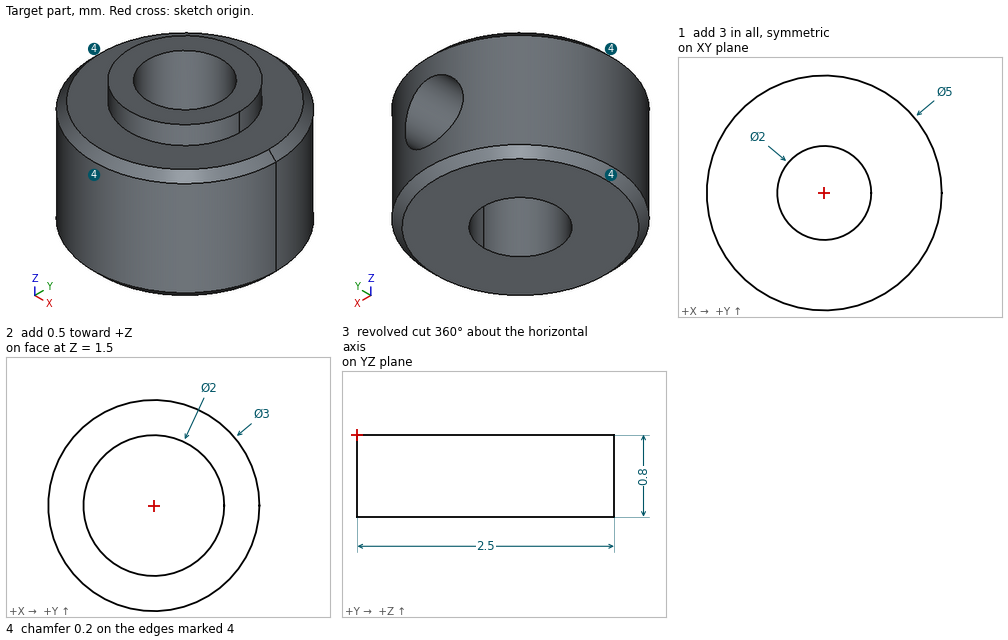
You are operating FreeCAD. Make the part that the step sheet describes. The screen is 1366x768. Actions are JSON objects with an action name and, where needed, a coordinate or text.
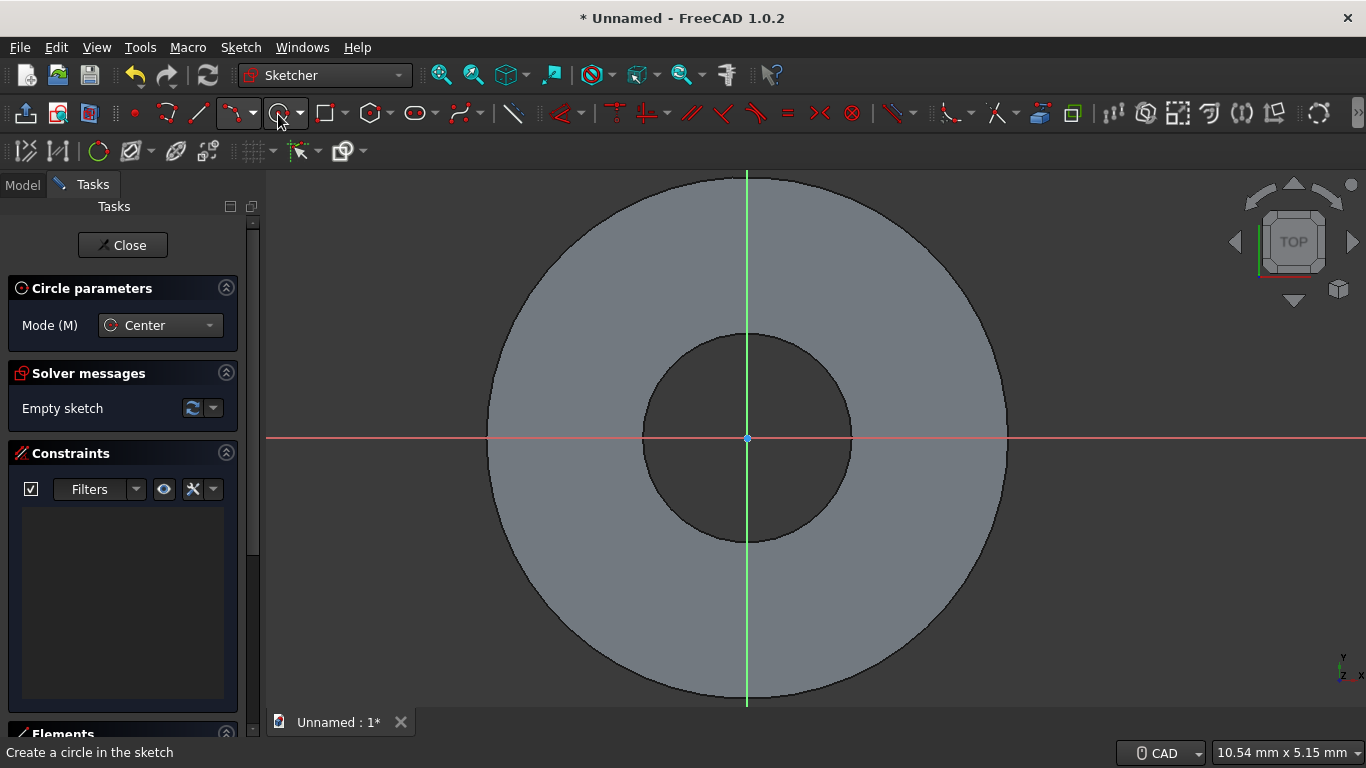
{"action": "left_click", "coordinate": [747, 438]}
{"action": "mouse_move", "coordinate": [858, 327]}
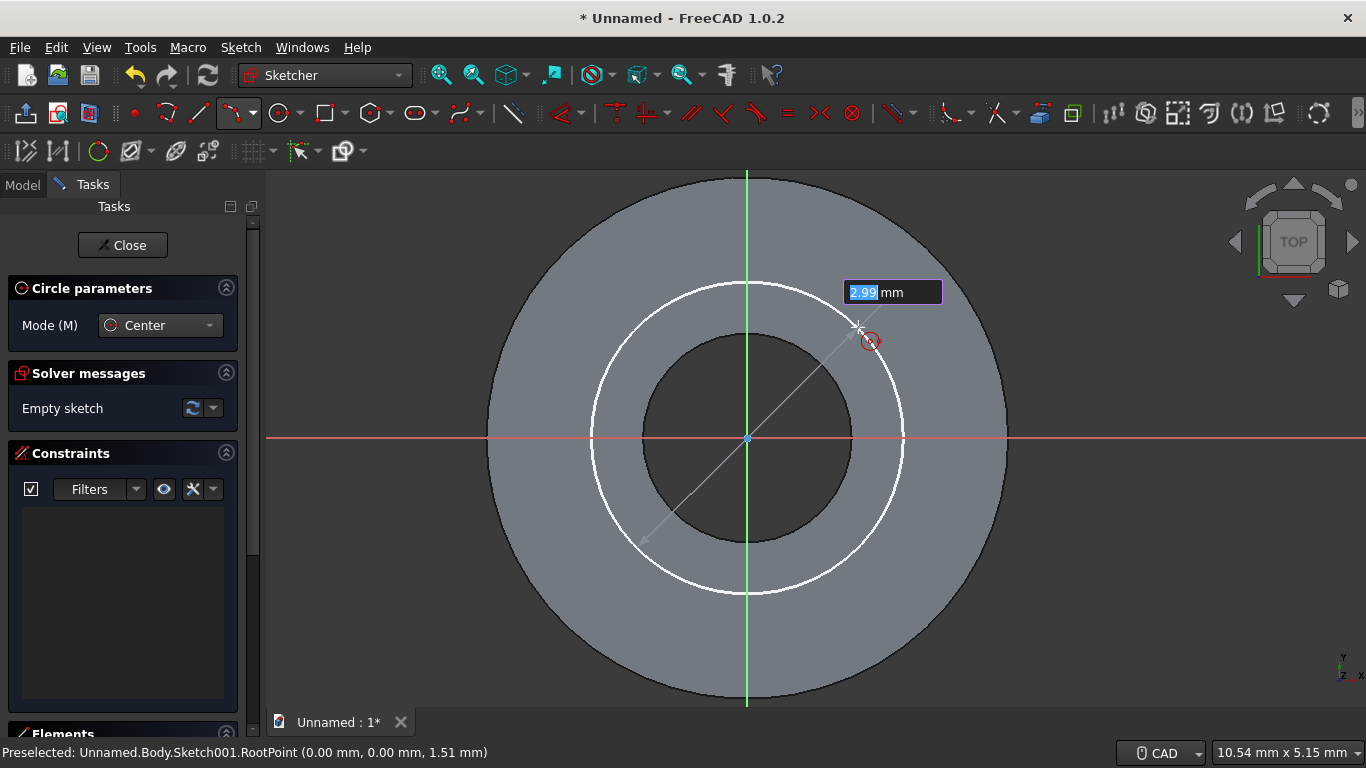
{"action": "type", "text": "3"}
{"action": "key", "text": "Return"}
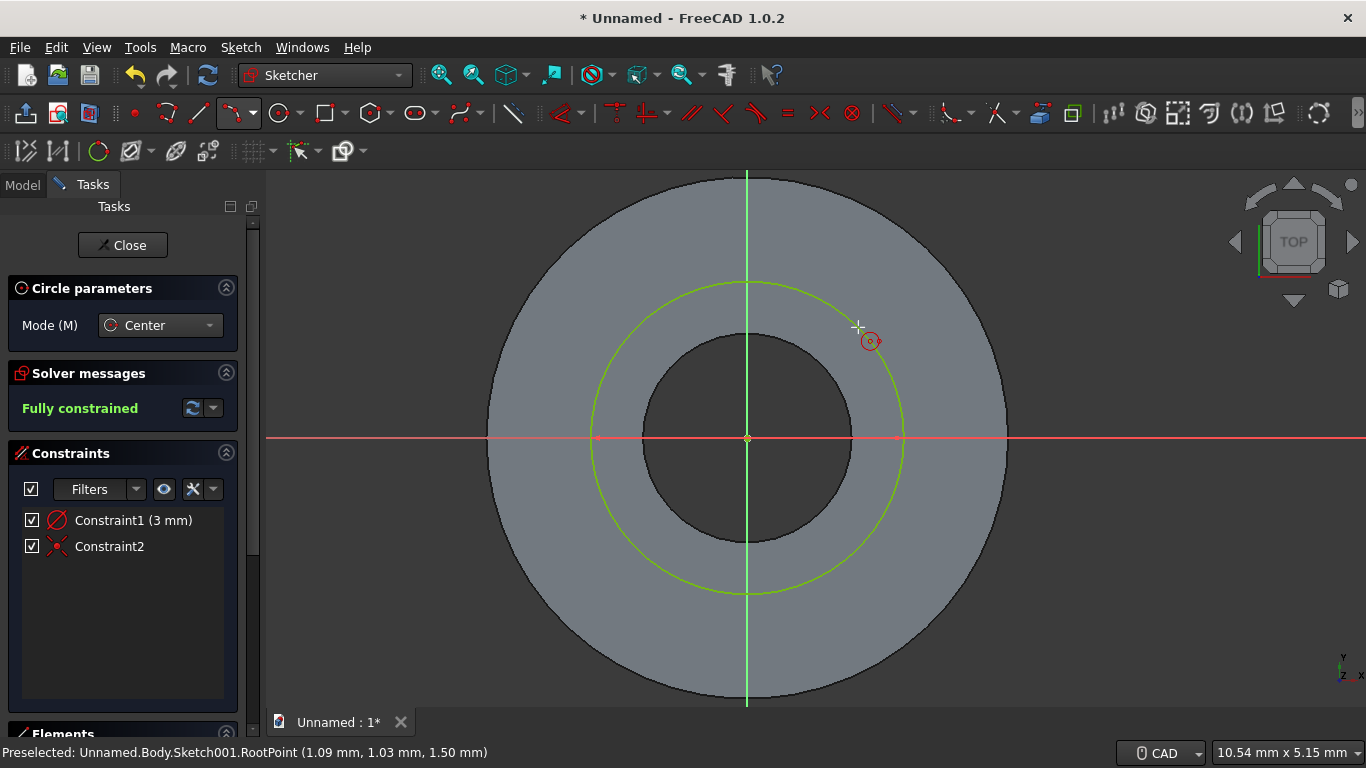
{"action": "left_click", "coordinate": [747, 438]}
{"action": "mouse_move", "coordinate": [821, 364]}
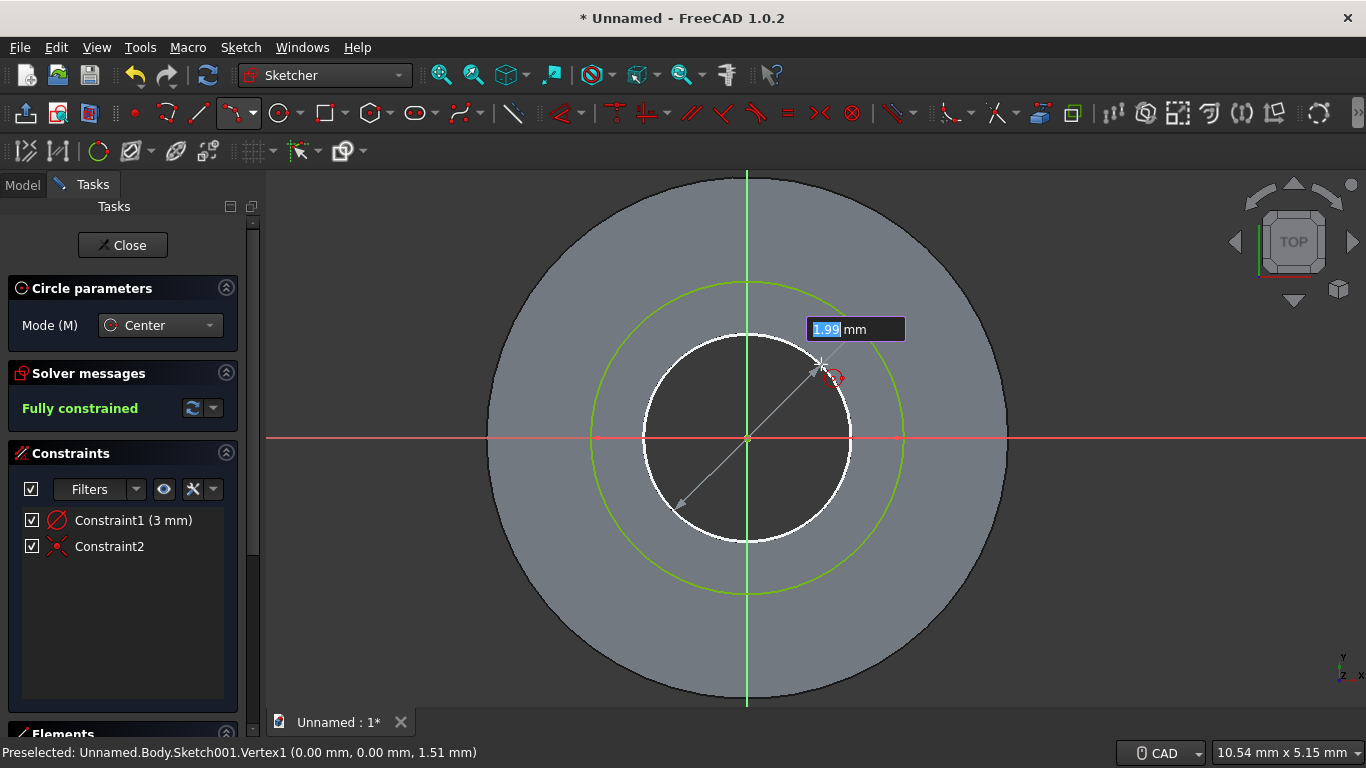
{"action": "type", "text": "2"}
{"action": "key", "text": "Return"}
{"action": "key", "text": "Escape"}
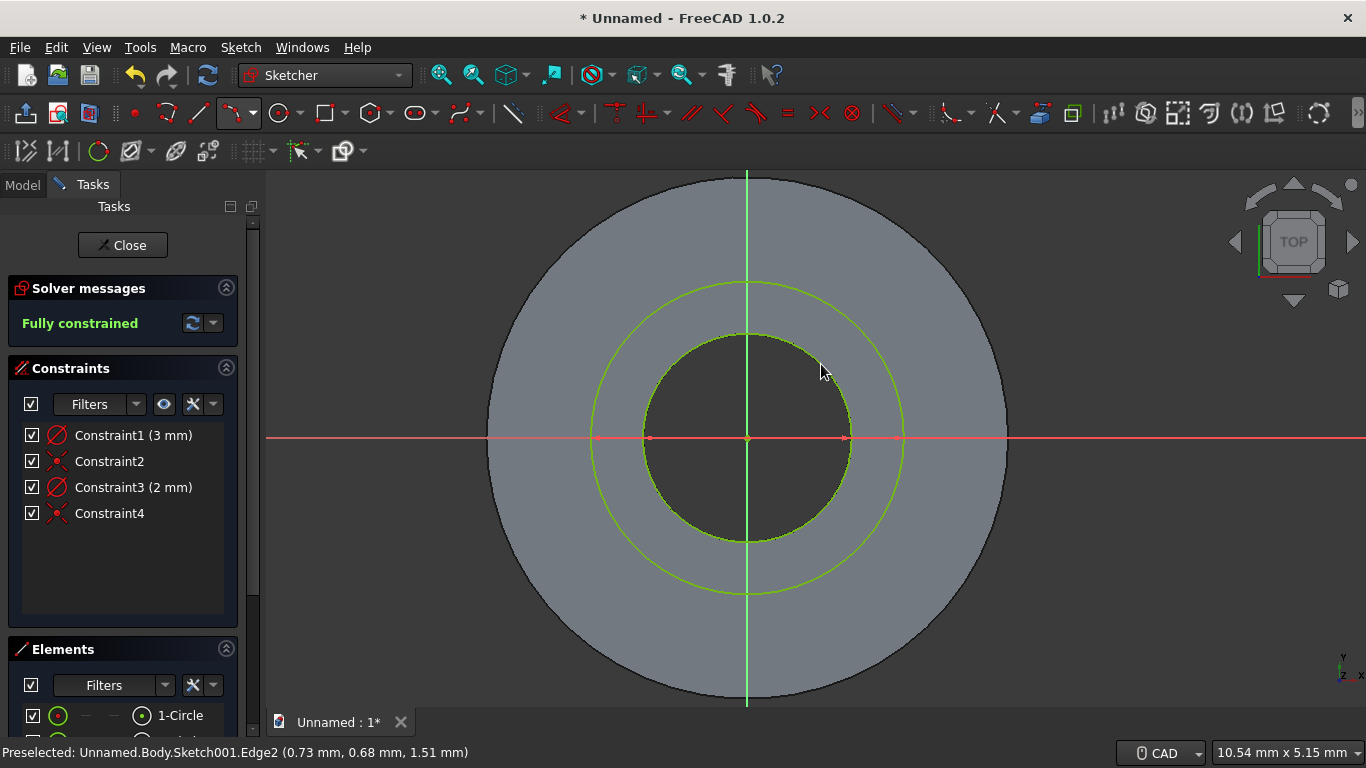
{"action": "left_click", "coordinate": [123, 245]}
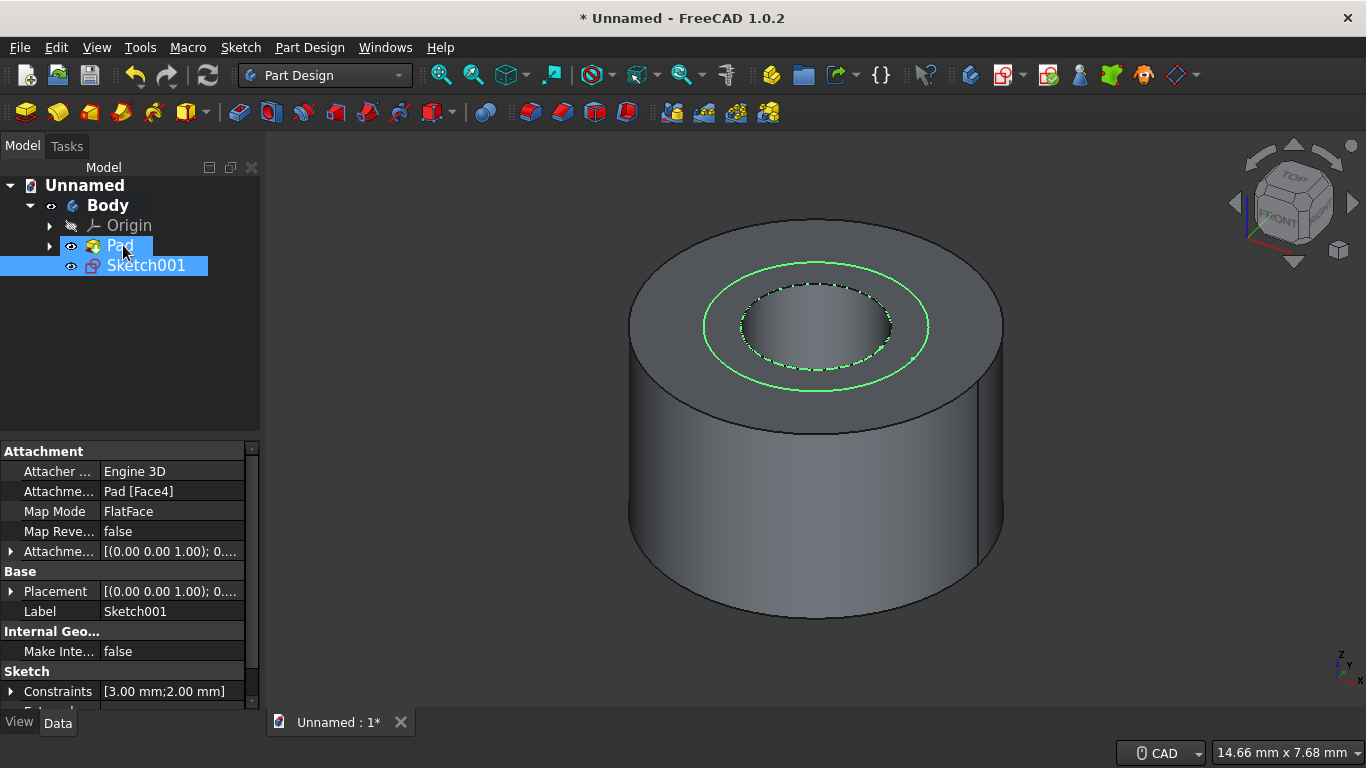
{"action": "left_click", "coordinate": [26, 112]}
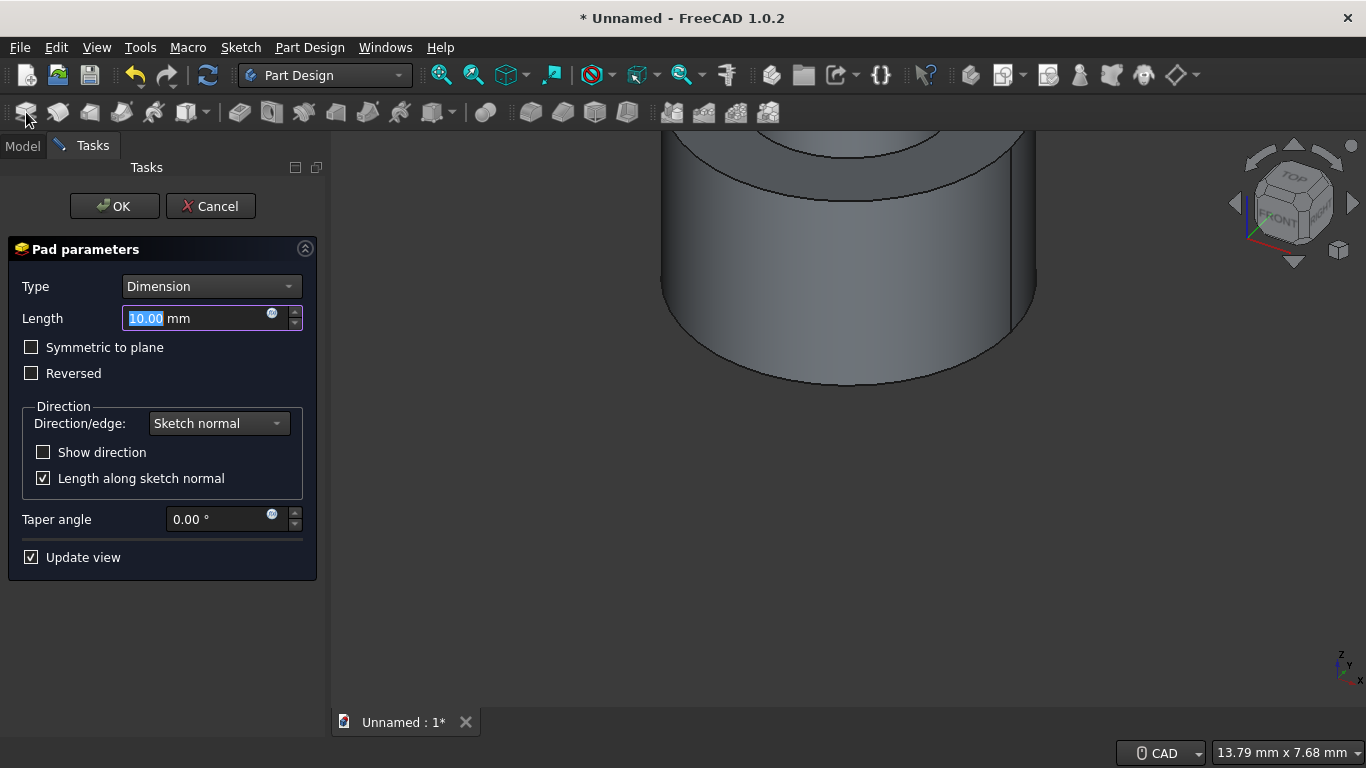
{"action": "type", "text": "0.5"}
{"action": "key", "text": "Tab"}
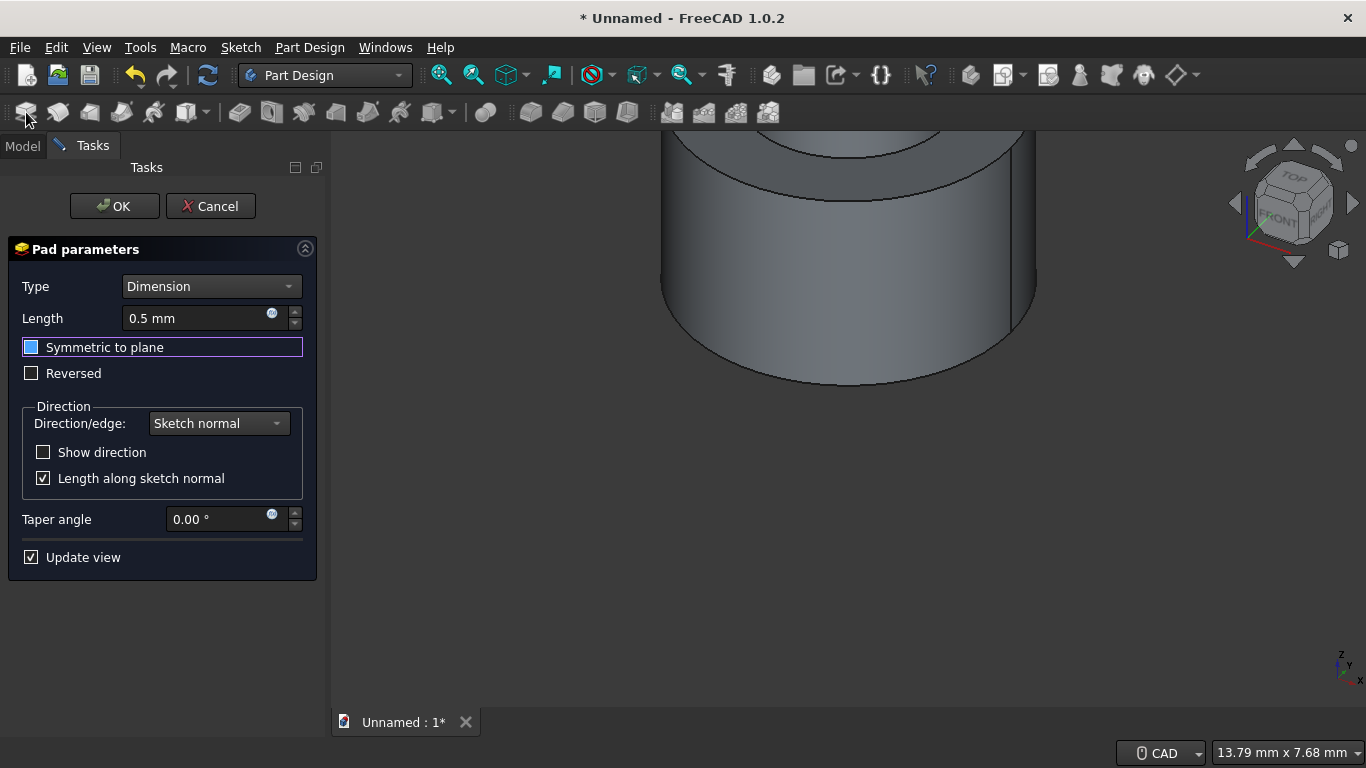
{"action": "left_click", "coordinate": [115, 206]}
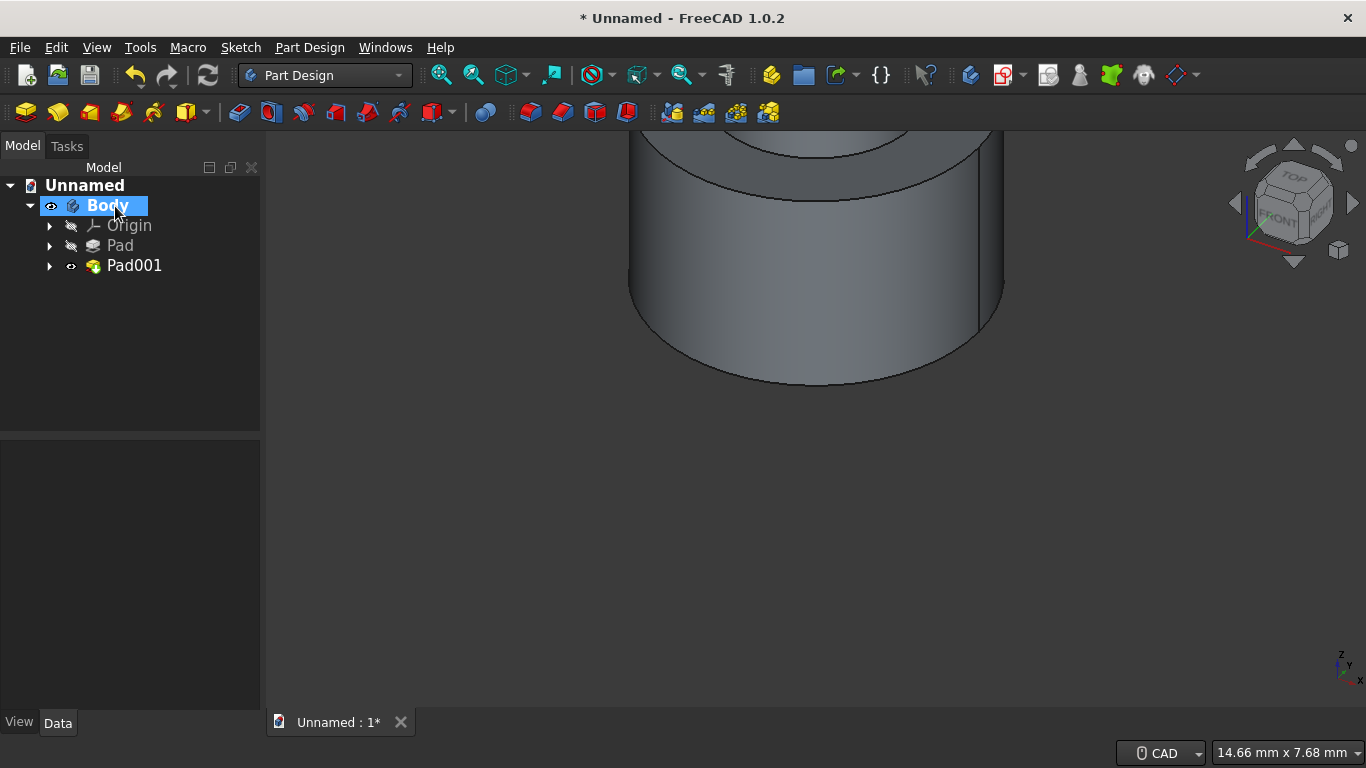
{"action": "left_click", "coordinate": [442, 76]}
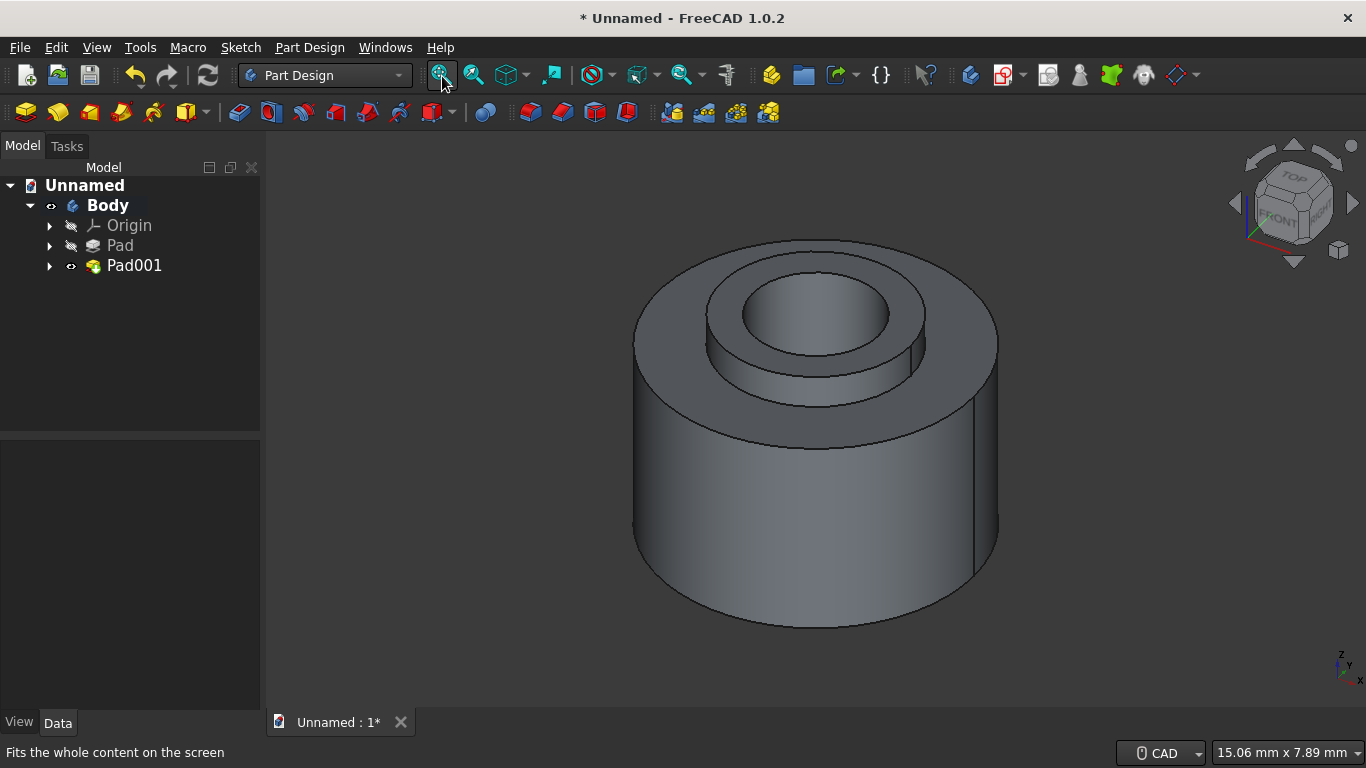
{"action": "left_click", "coordinate": [1004, 76]}